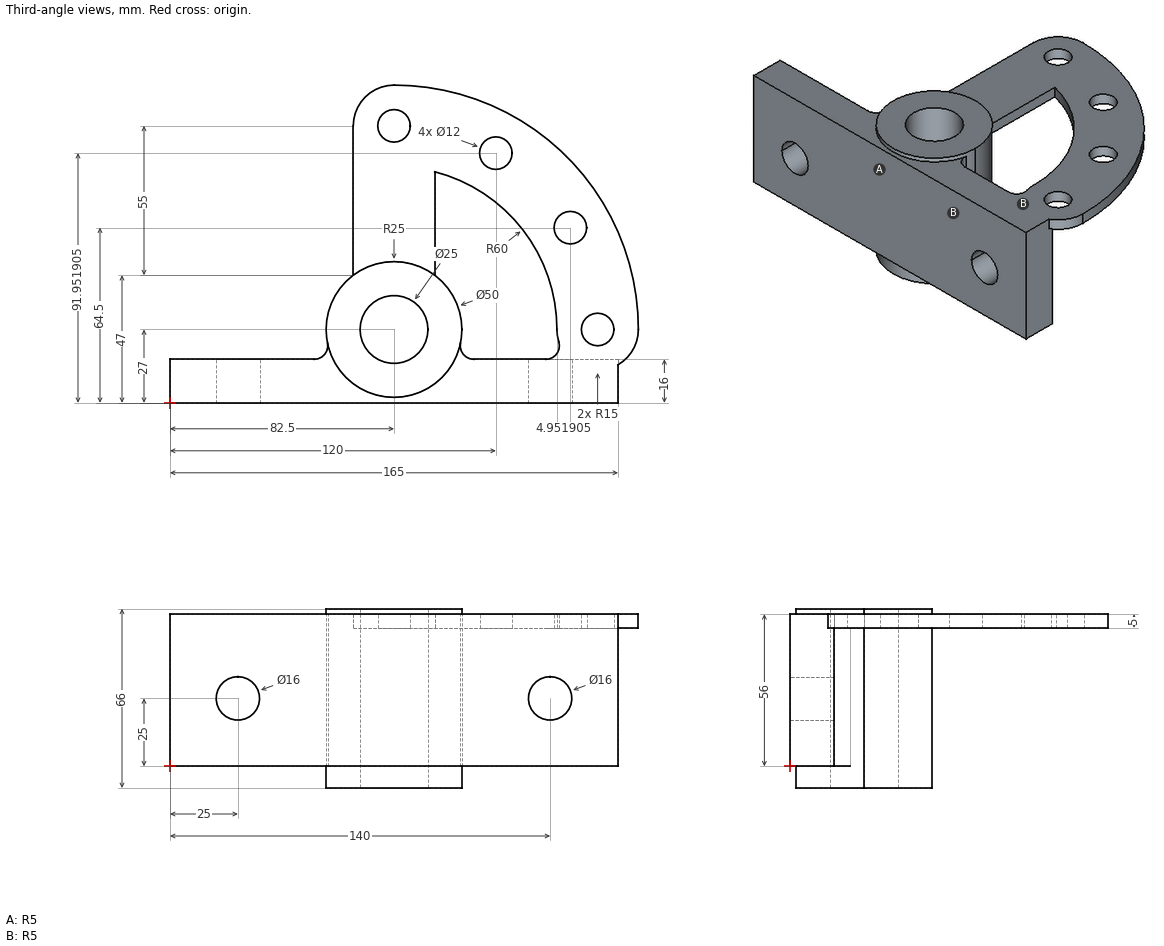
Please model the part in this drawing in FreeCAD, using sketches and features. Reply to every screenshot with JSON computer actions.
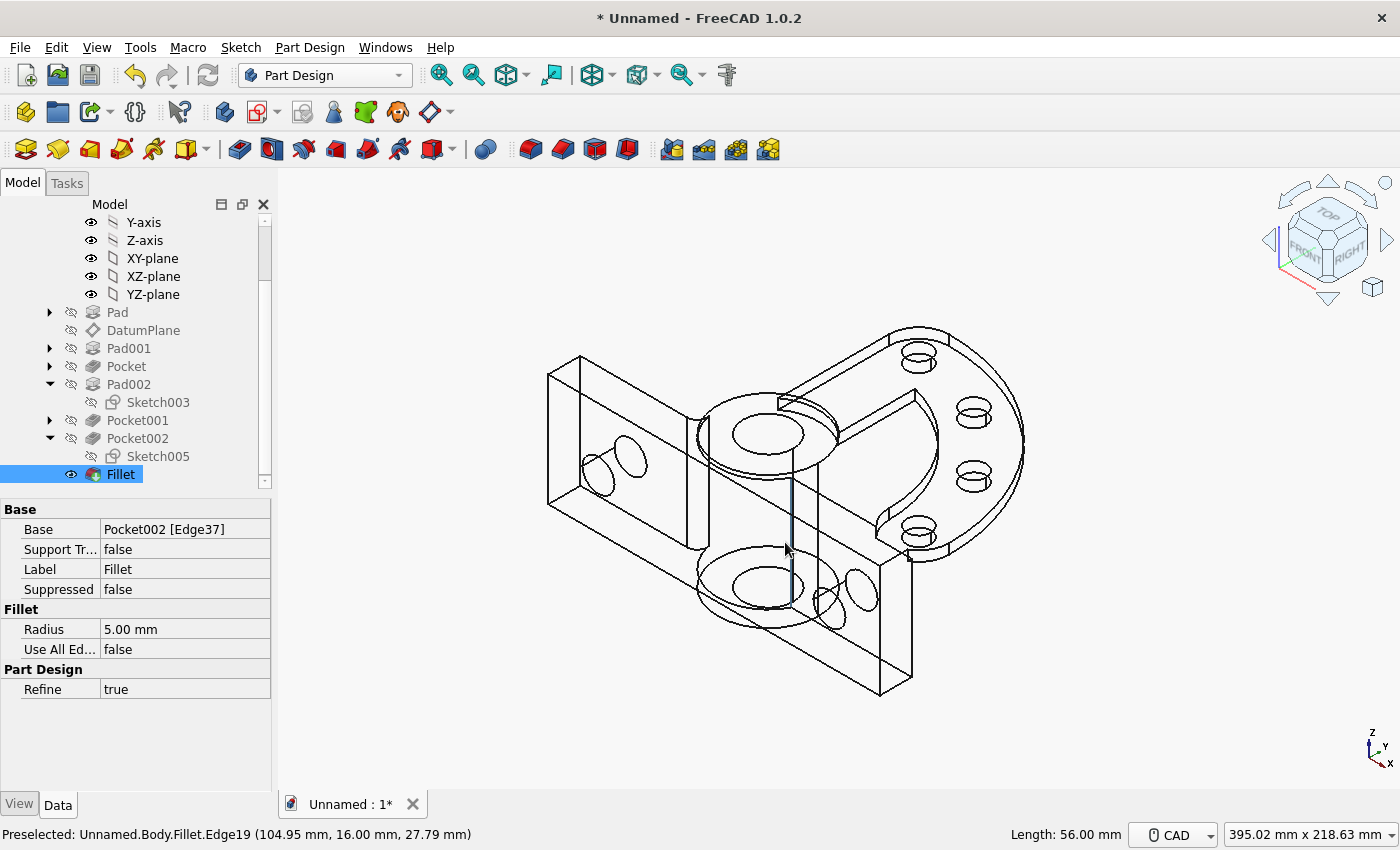
{"action": "left_click", "coordinate": [876, 533], "text": "ctrl"}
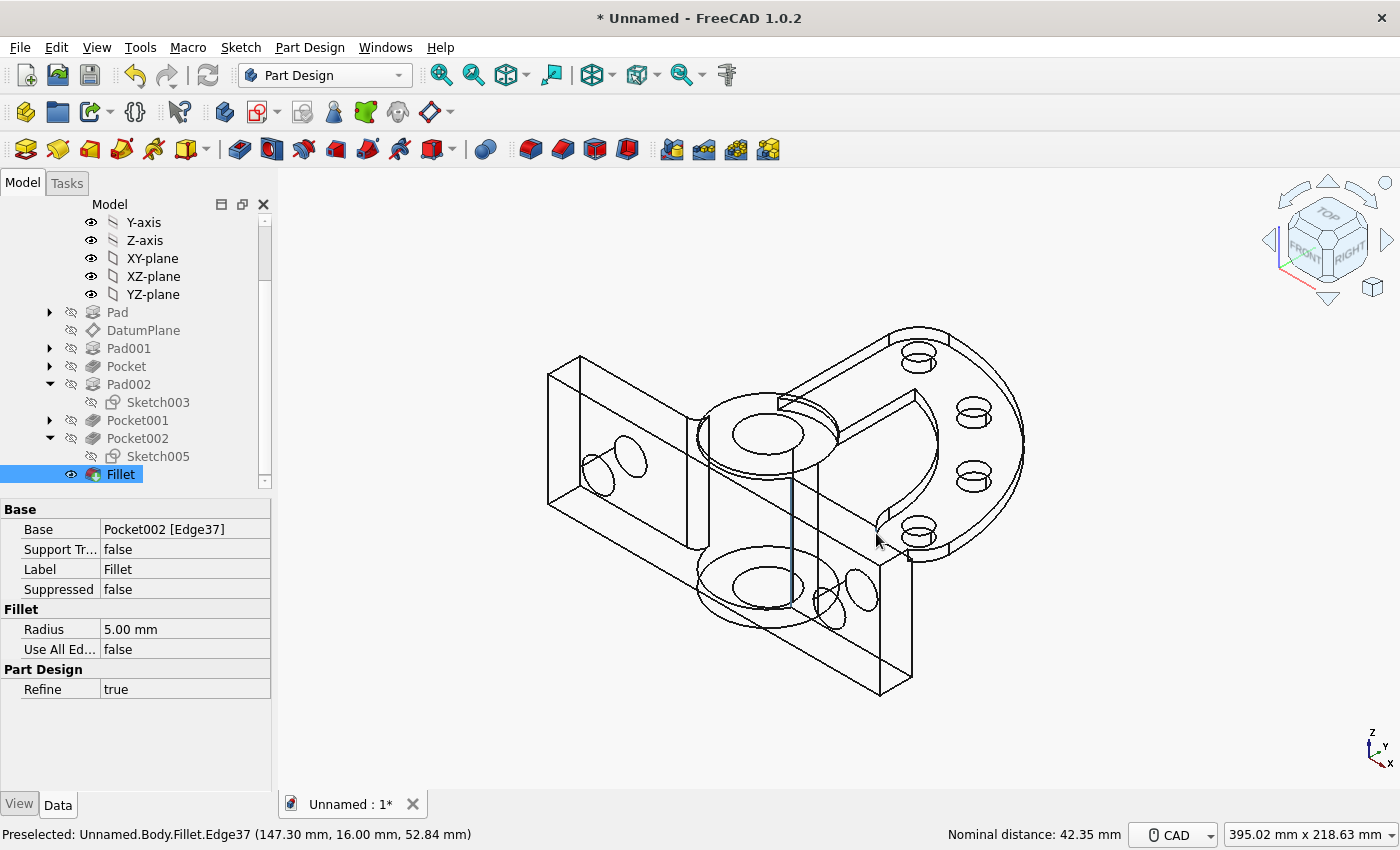
{"action": "key", "text": "v 1"}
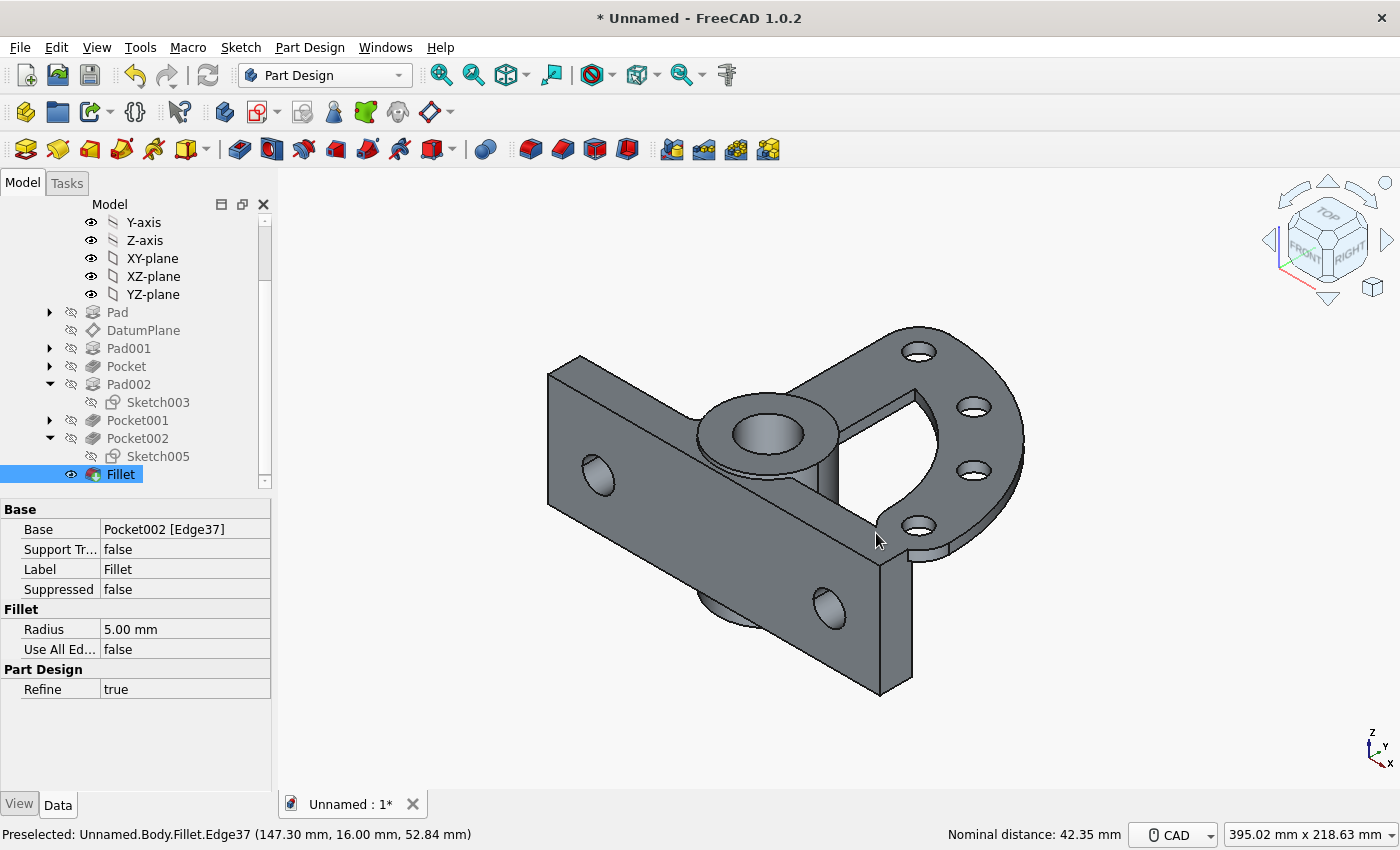
{"action": "left_click", "coordinate": [532, 150]}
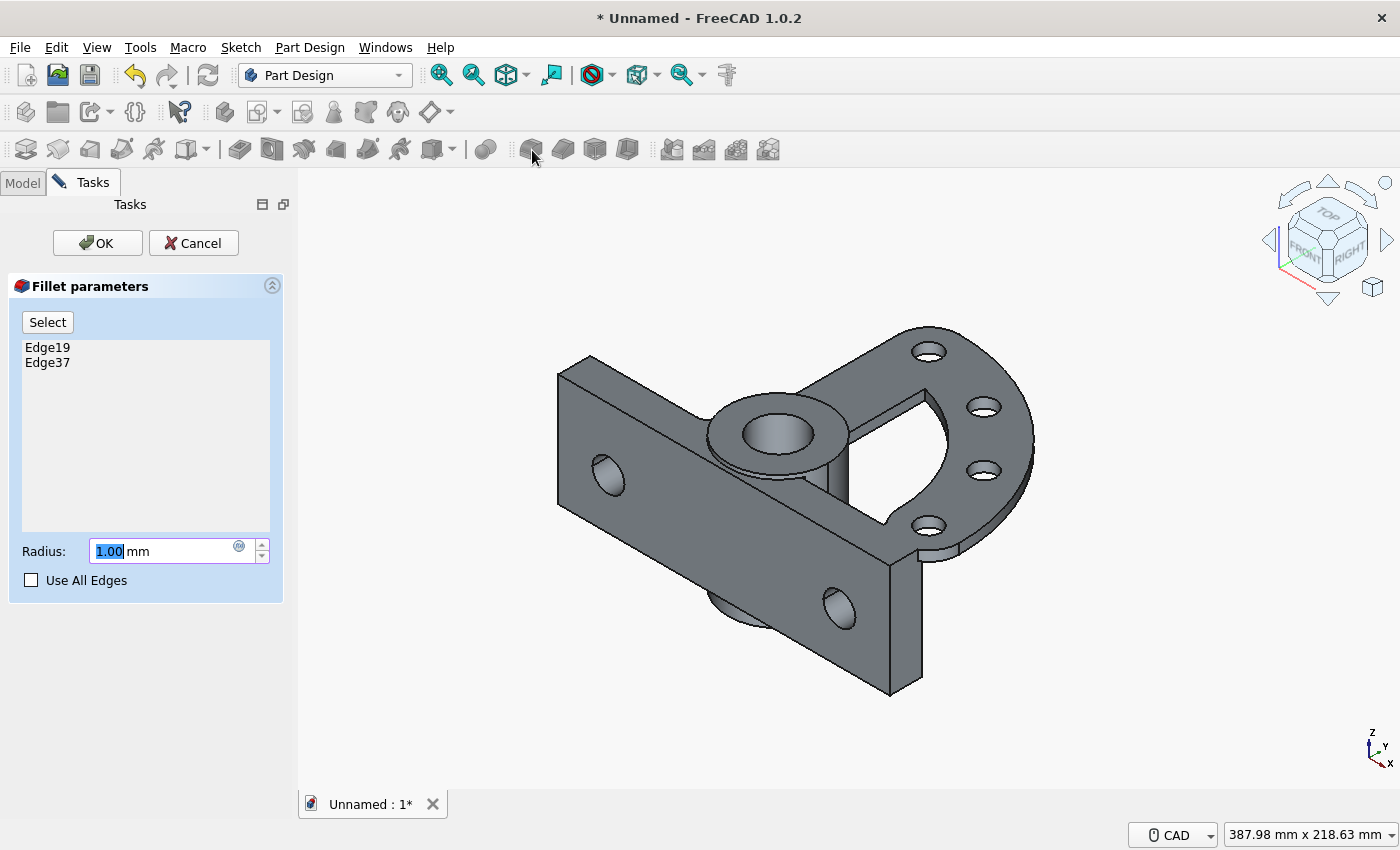
{"action": "type", "text": "5"}
{"action": "key", "text": "Tab"}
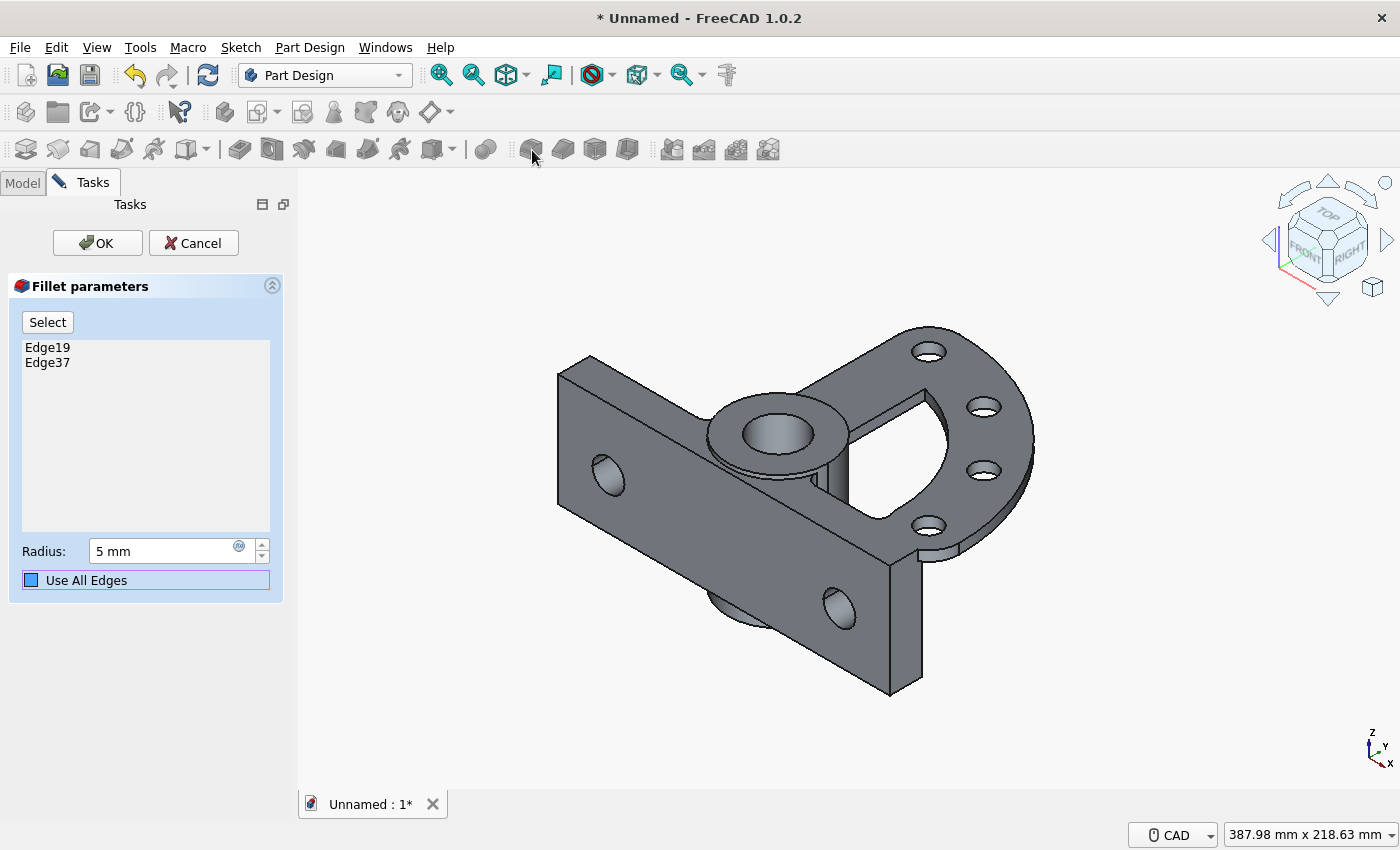
{"action": "left_click", "coordinate": [98, 243]}